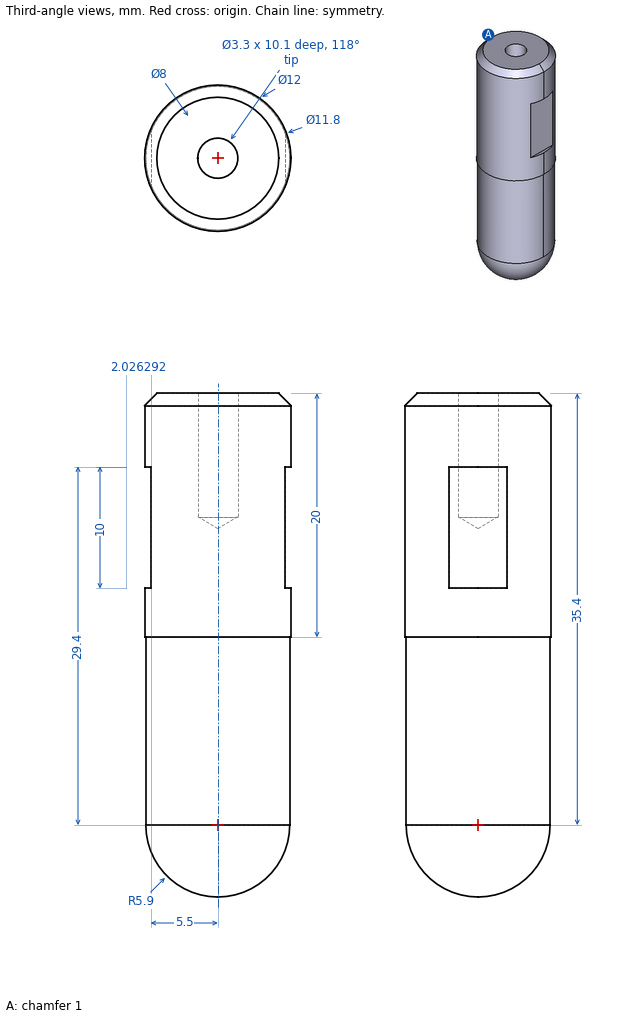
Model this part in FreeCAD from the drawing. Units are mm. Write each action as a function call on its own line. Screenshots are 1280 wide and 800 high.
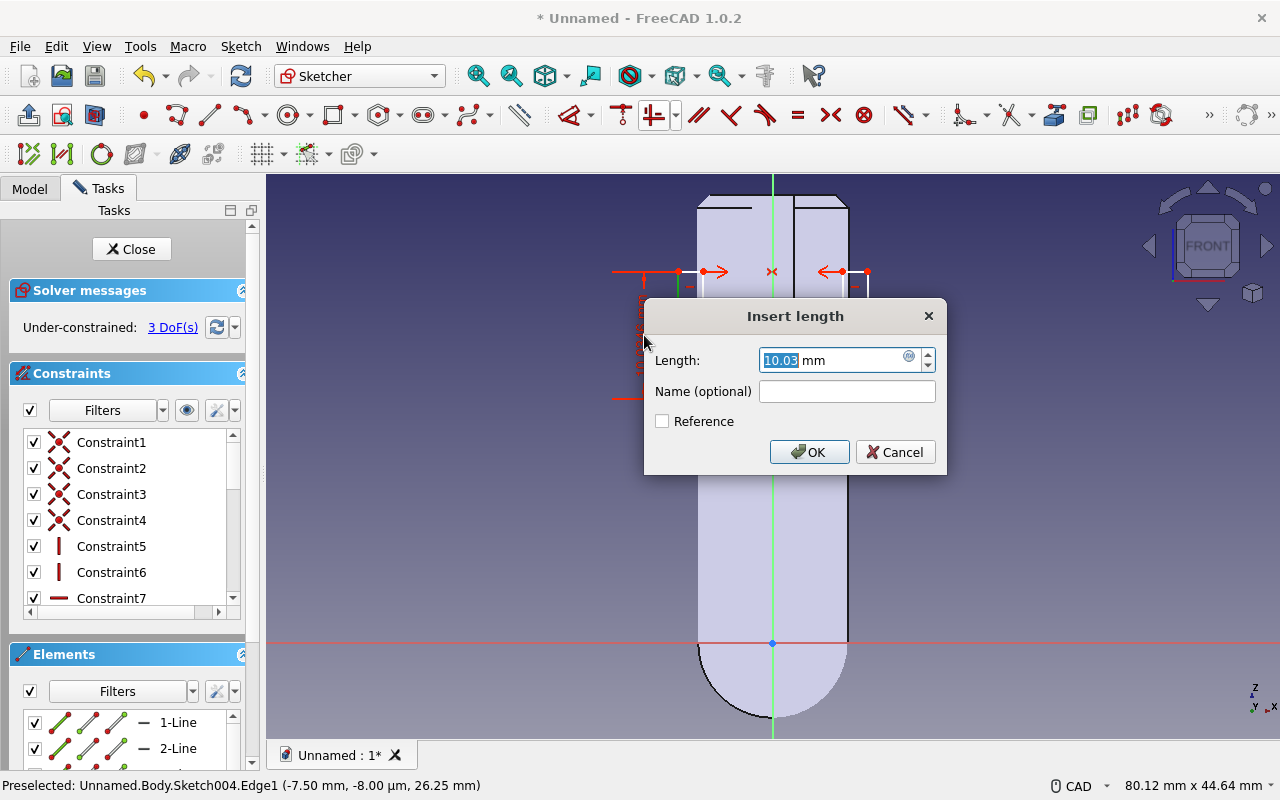
text(10)
key(Return)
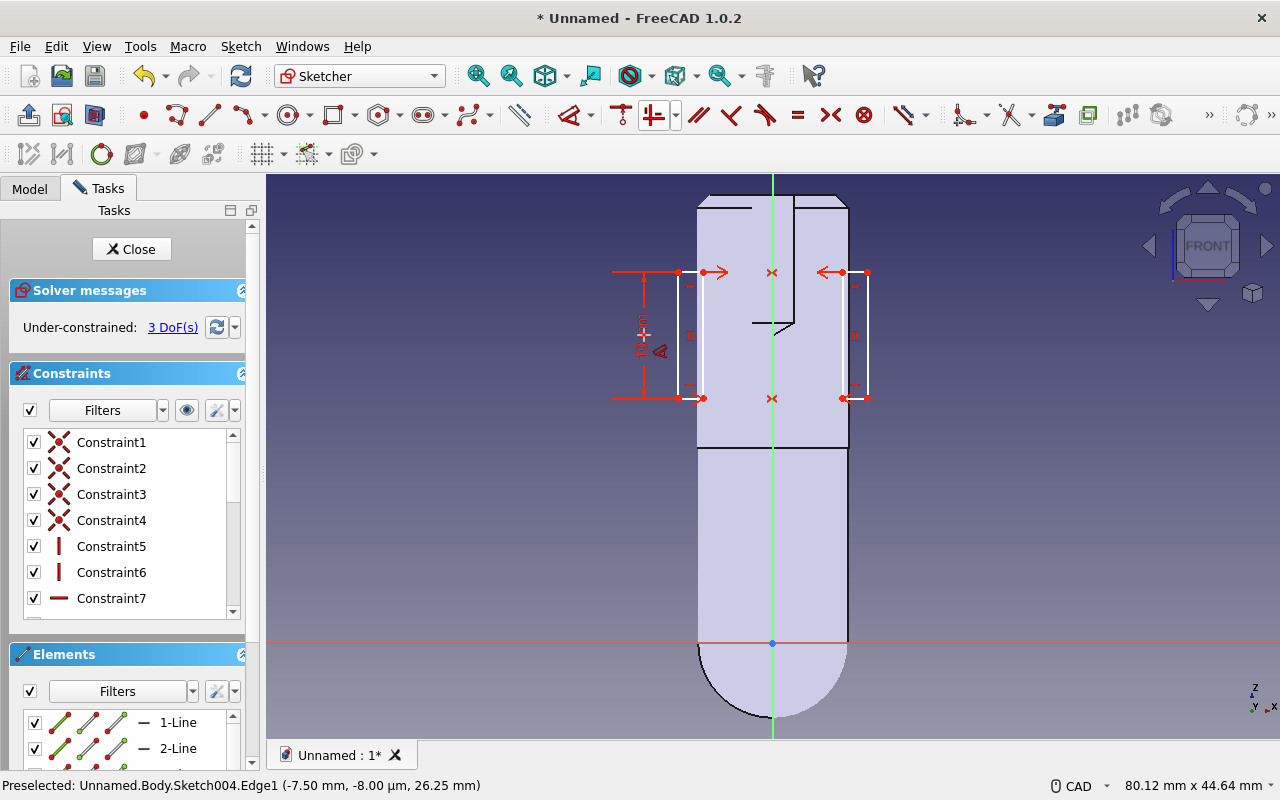
click(703, 399)
click(738, 677)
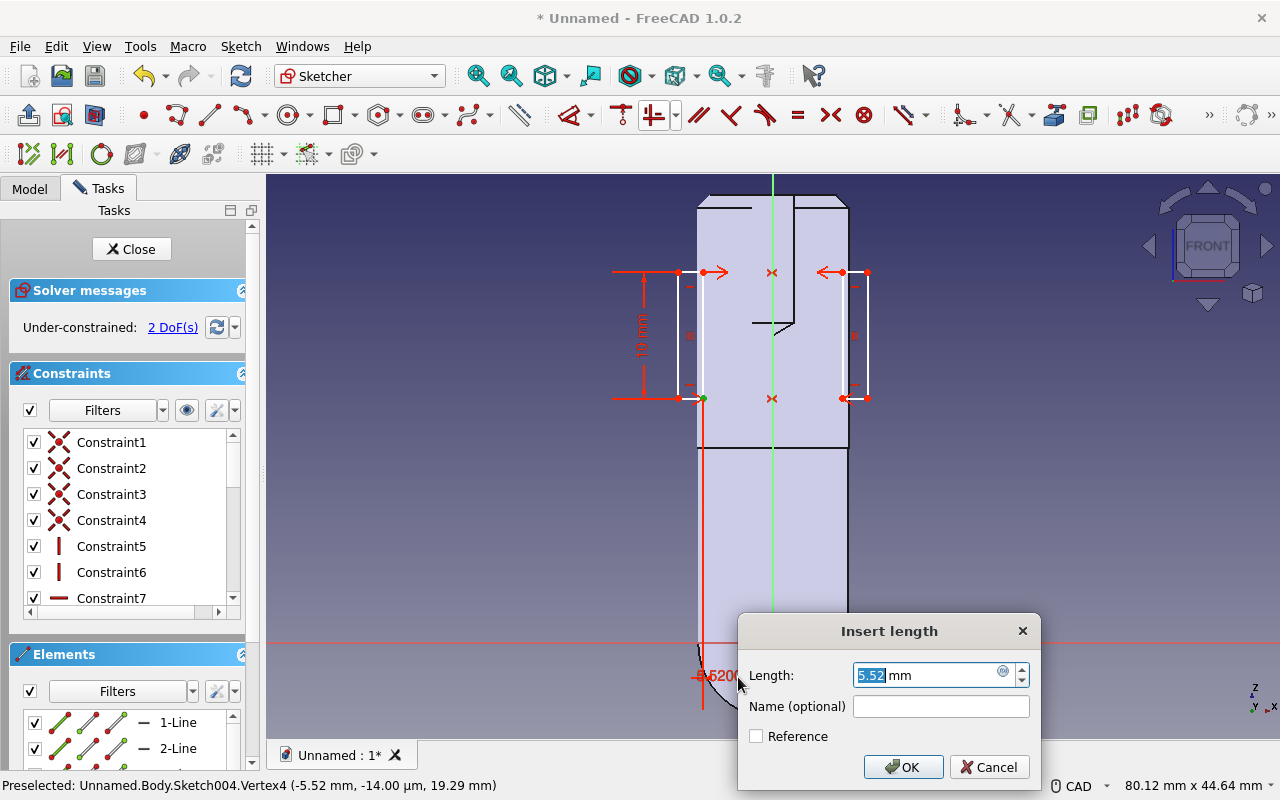
text(5.5)
key(Return)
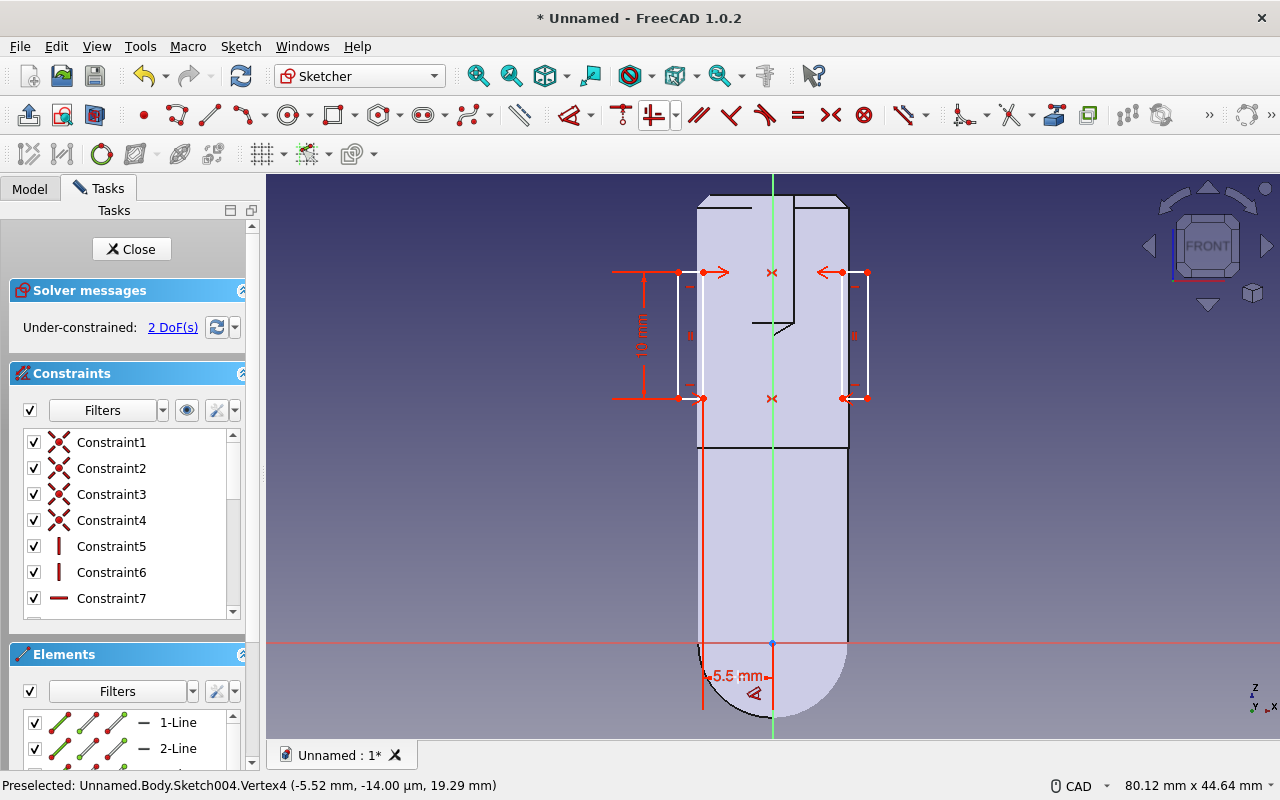
click(678, 272)
click(644, 458)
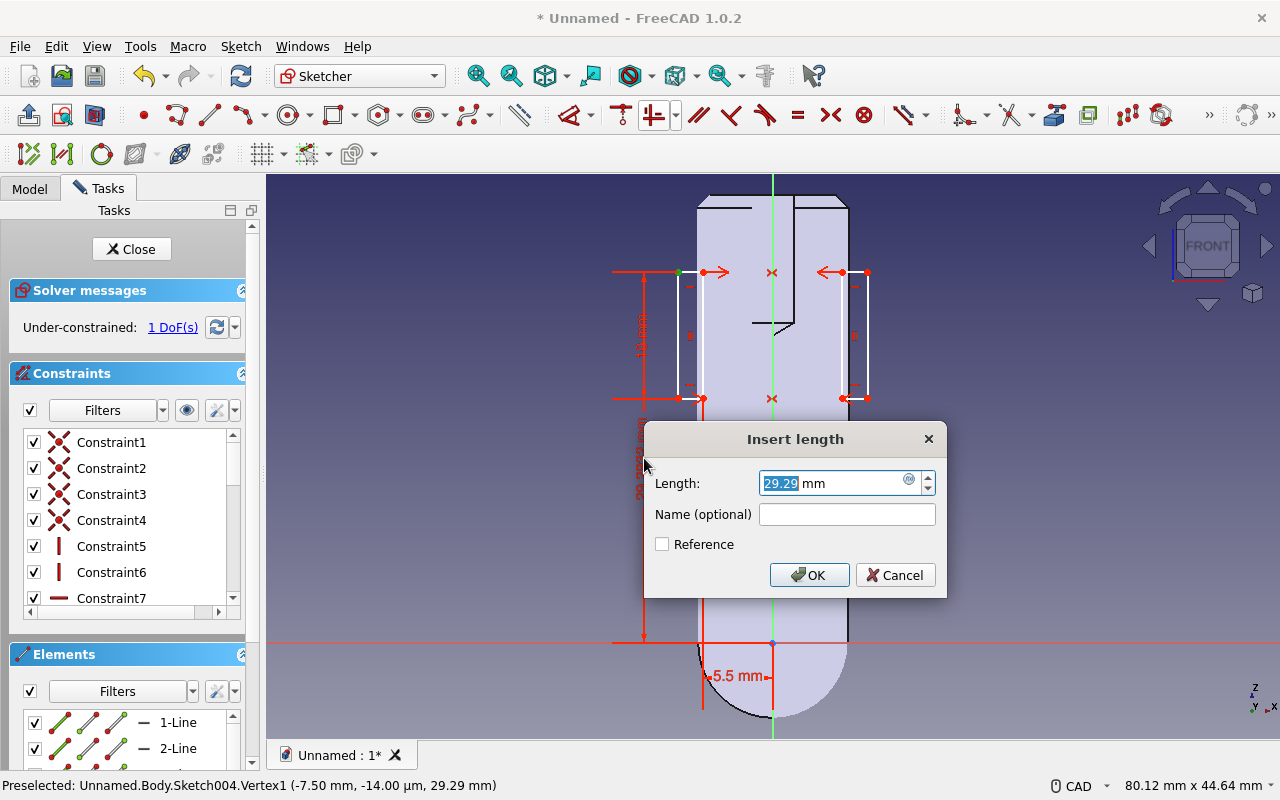
text(29.4)
key(Return)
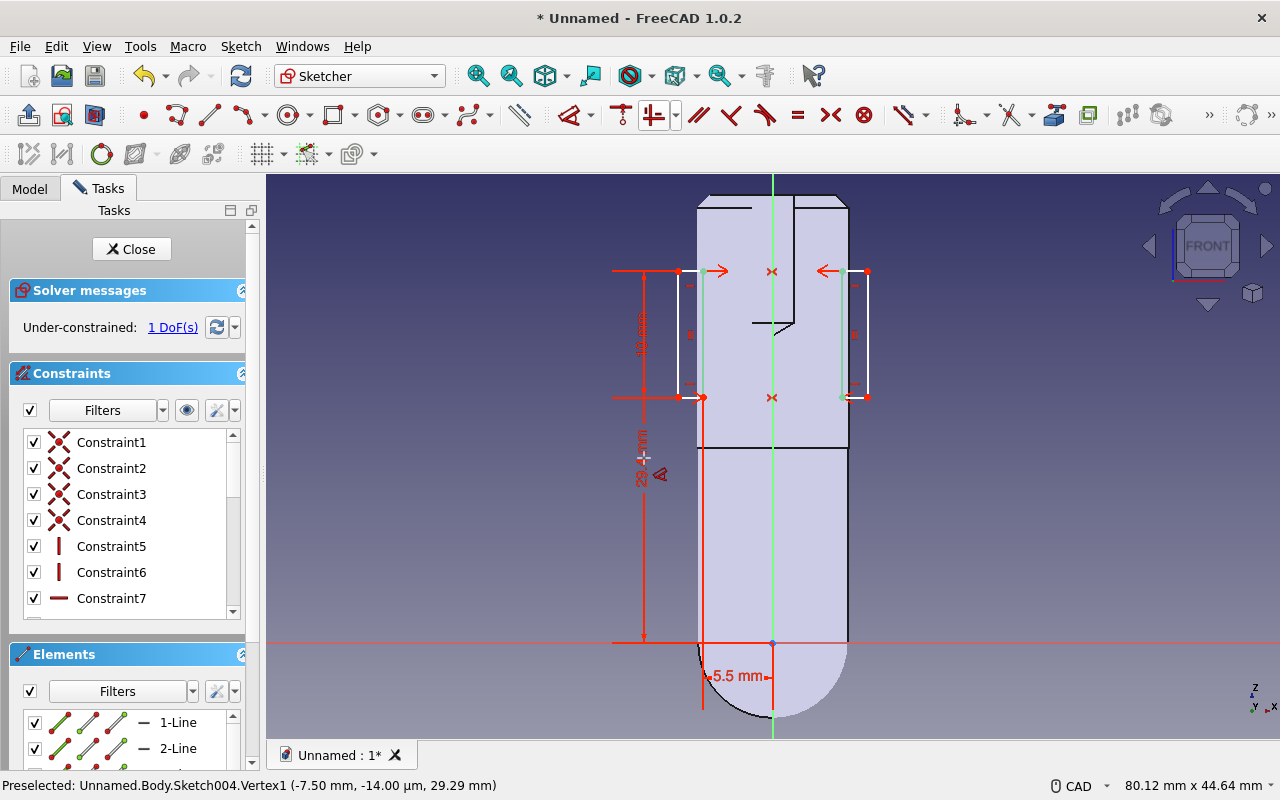
scroll(688, 398, up, 3)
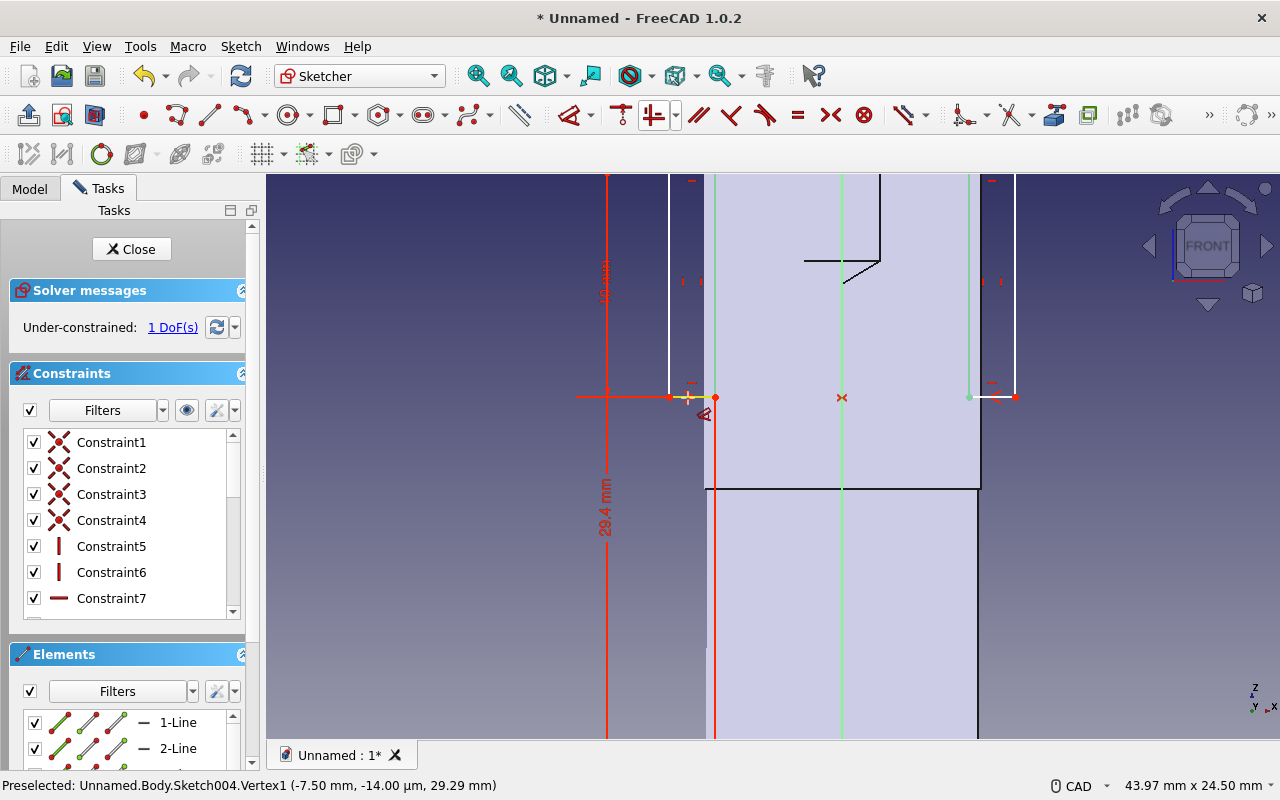
click(688, 397)
click(692, 363)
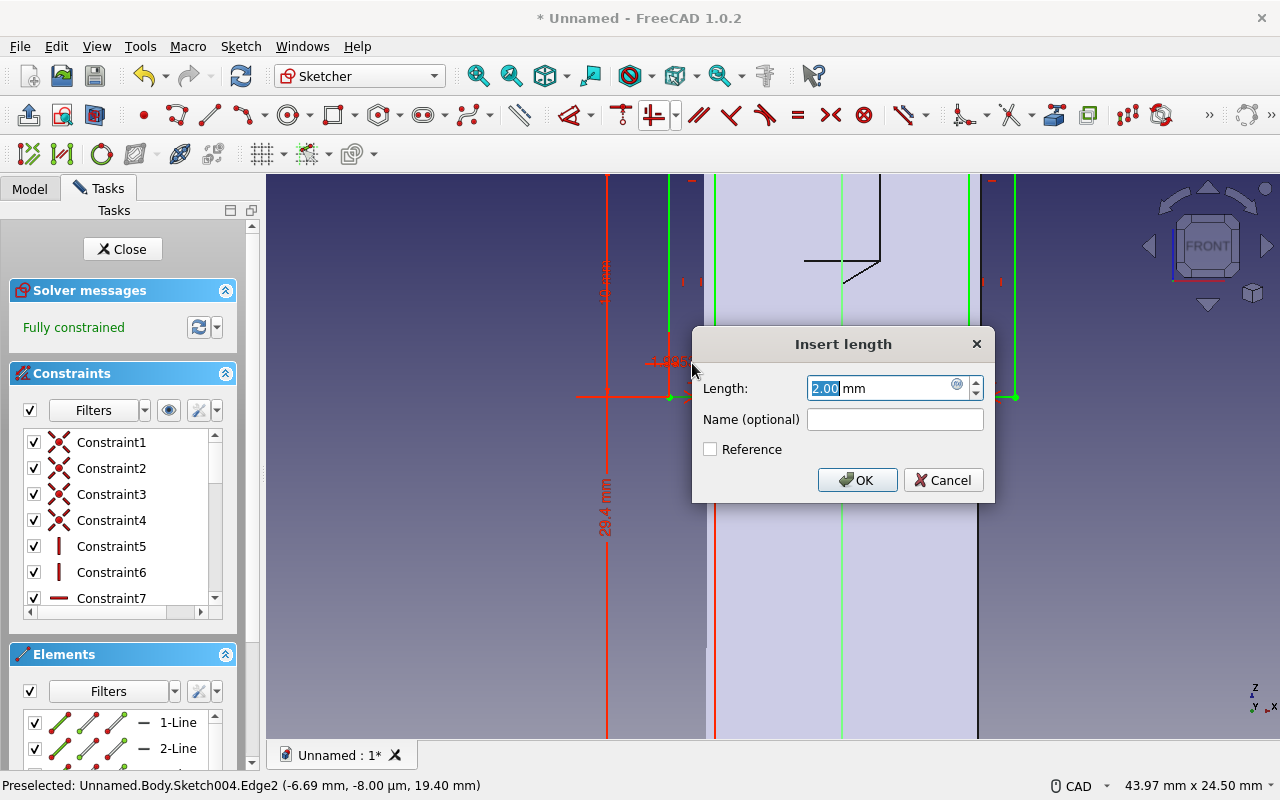
text(2.026292)
key(Return)
key(Escape)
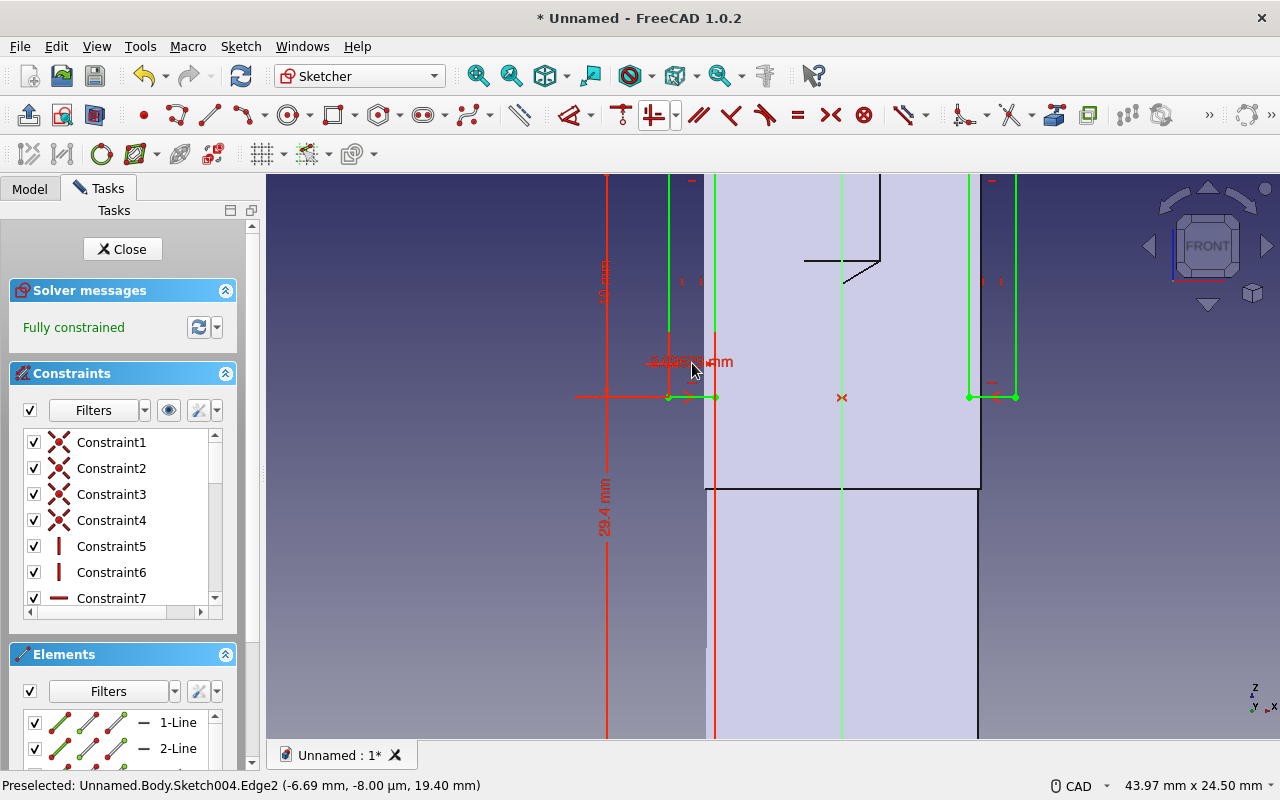
click(123, 249)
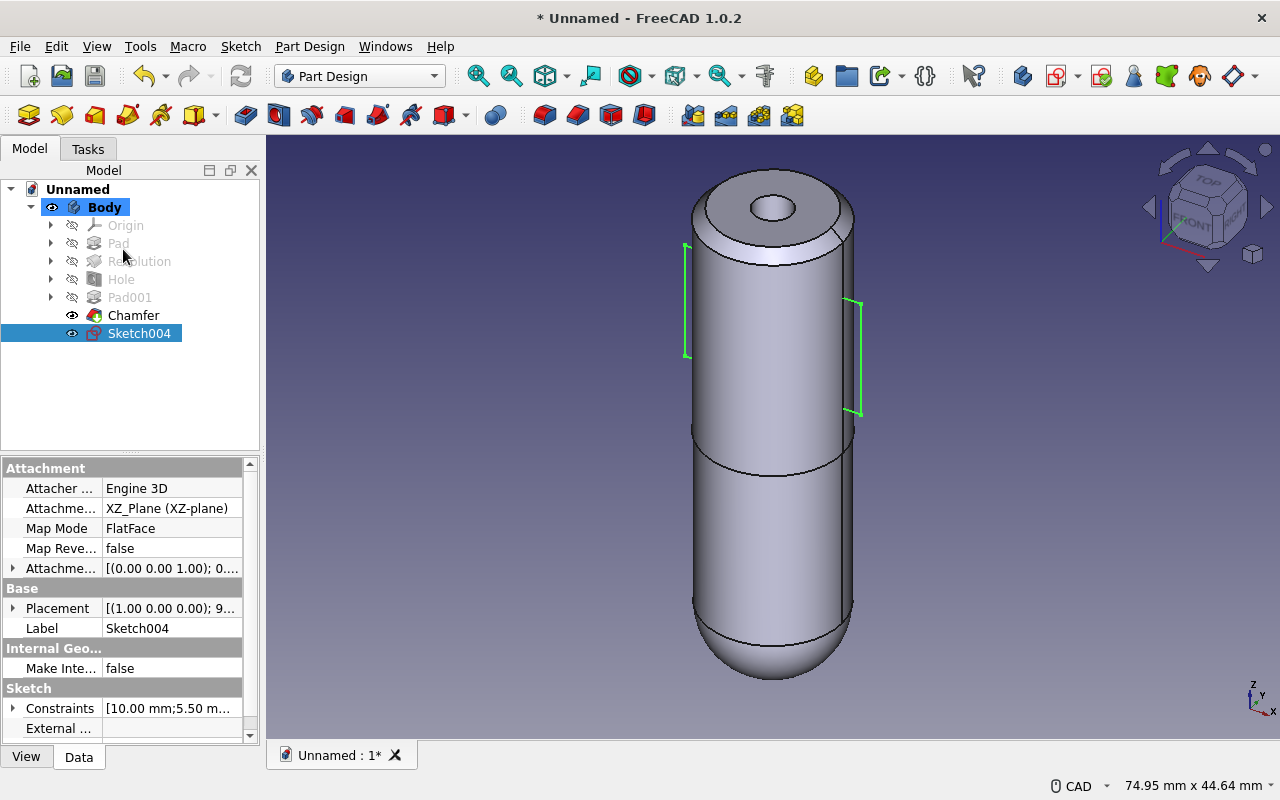
click(246, 116)